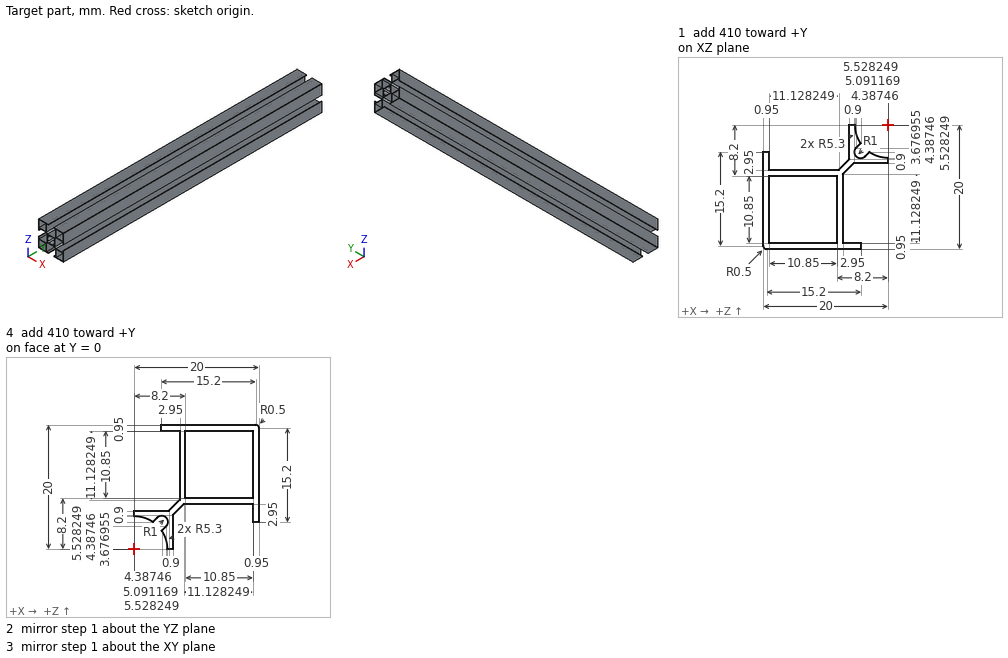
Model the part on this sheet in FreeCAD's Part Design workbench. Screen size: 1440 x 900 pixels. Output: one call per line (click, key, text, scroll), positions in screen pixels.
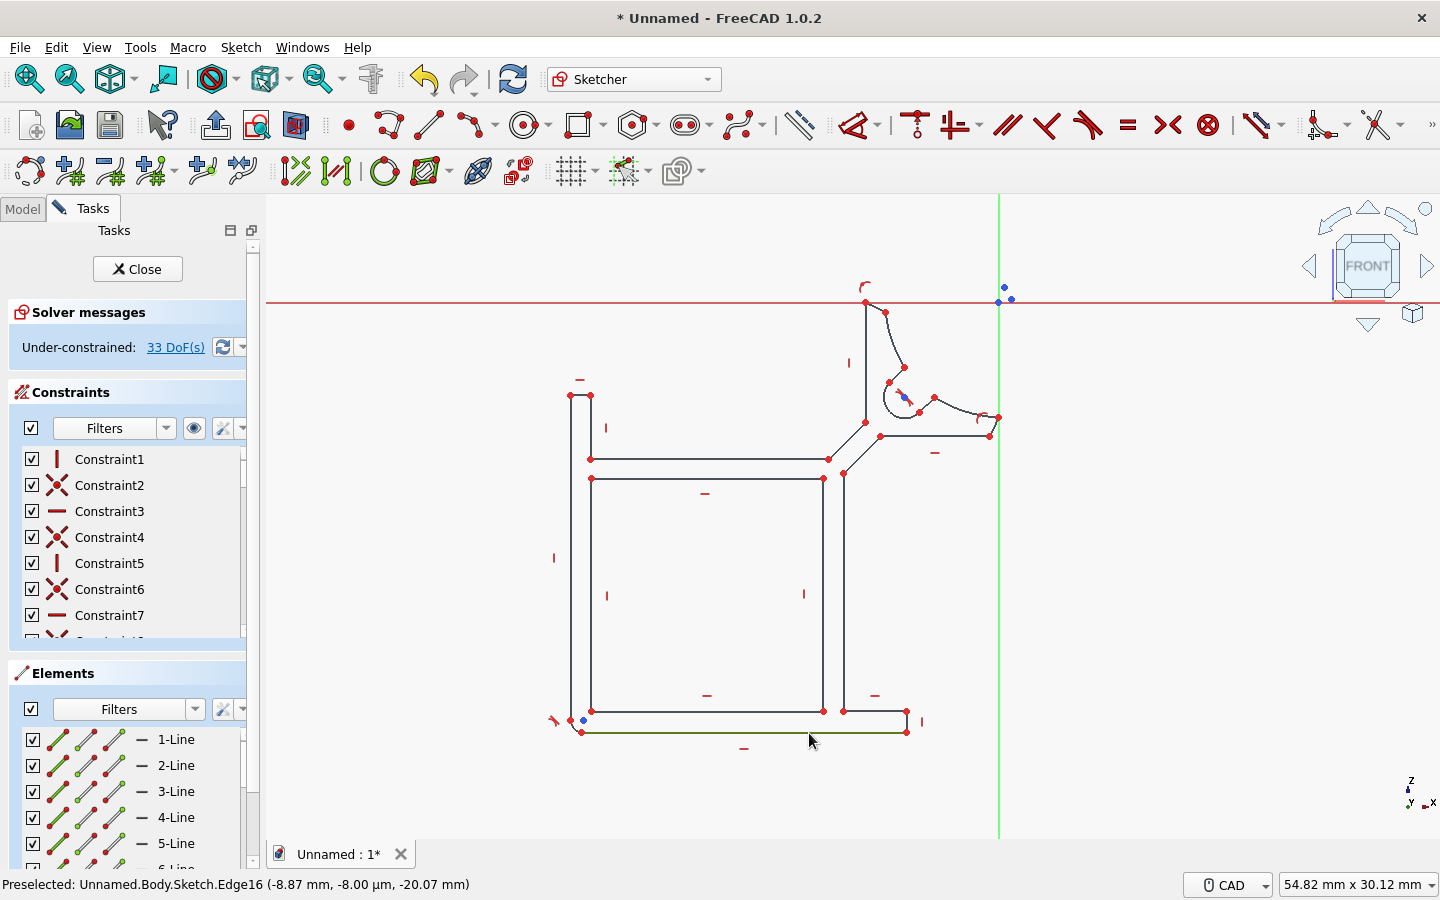
scroll(574, 728, up, 3)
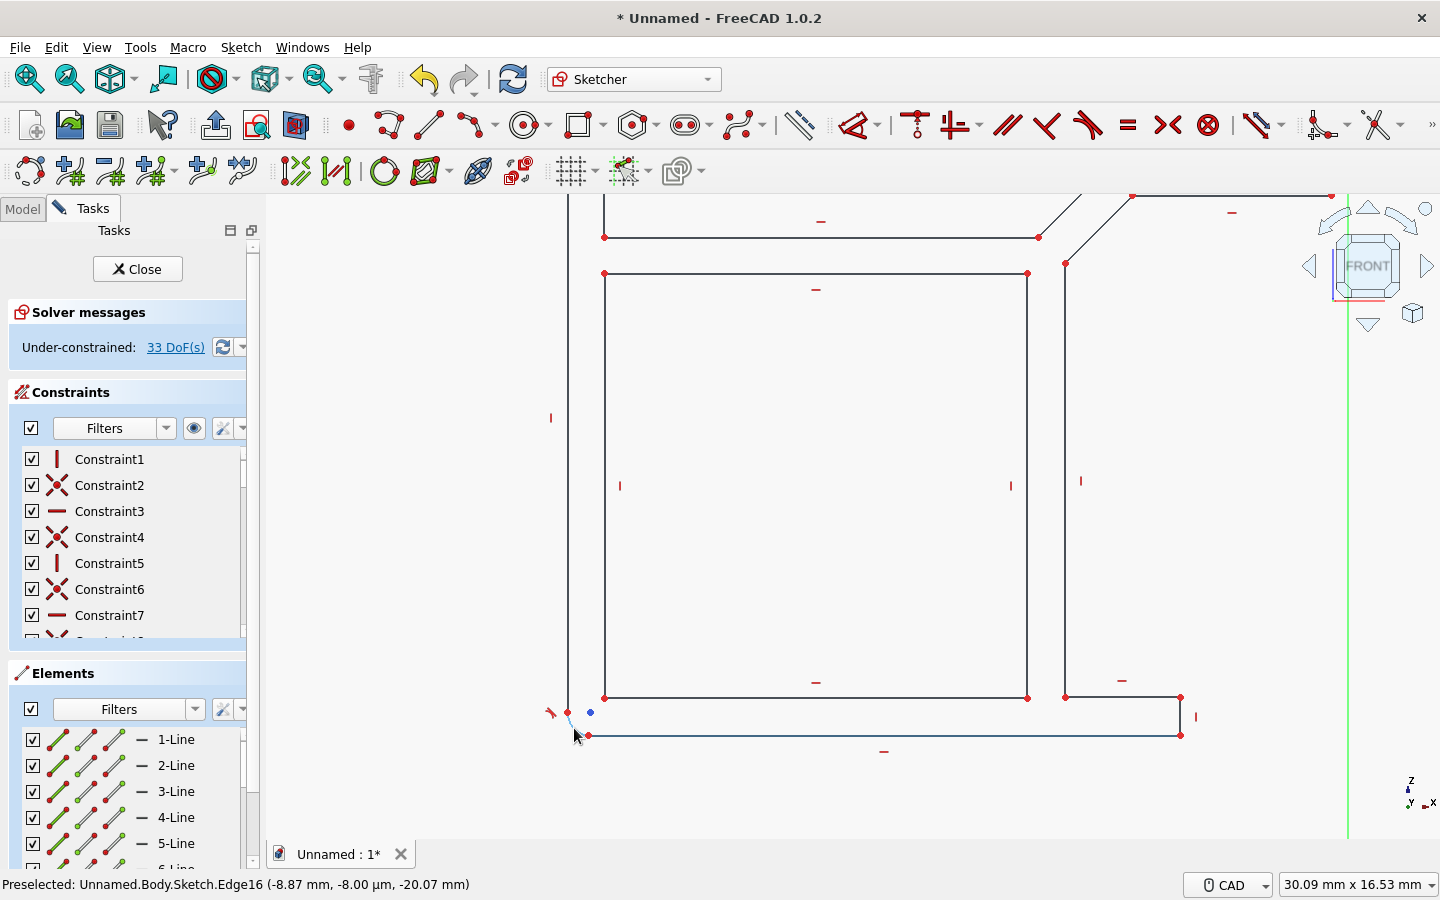
click(574, 728)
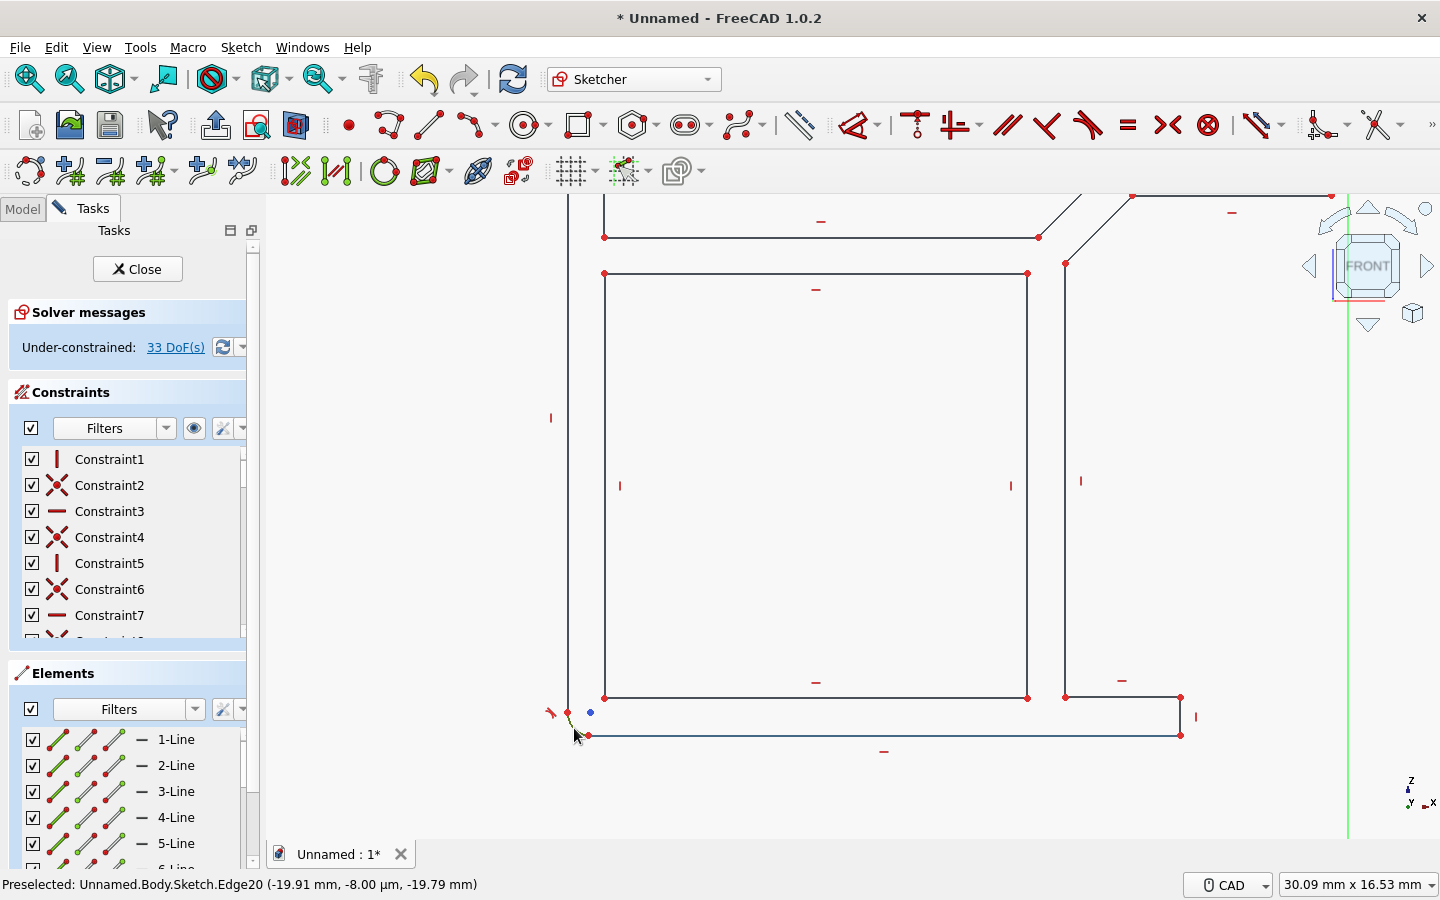
click(1088, 126)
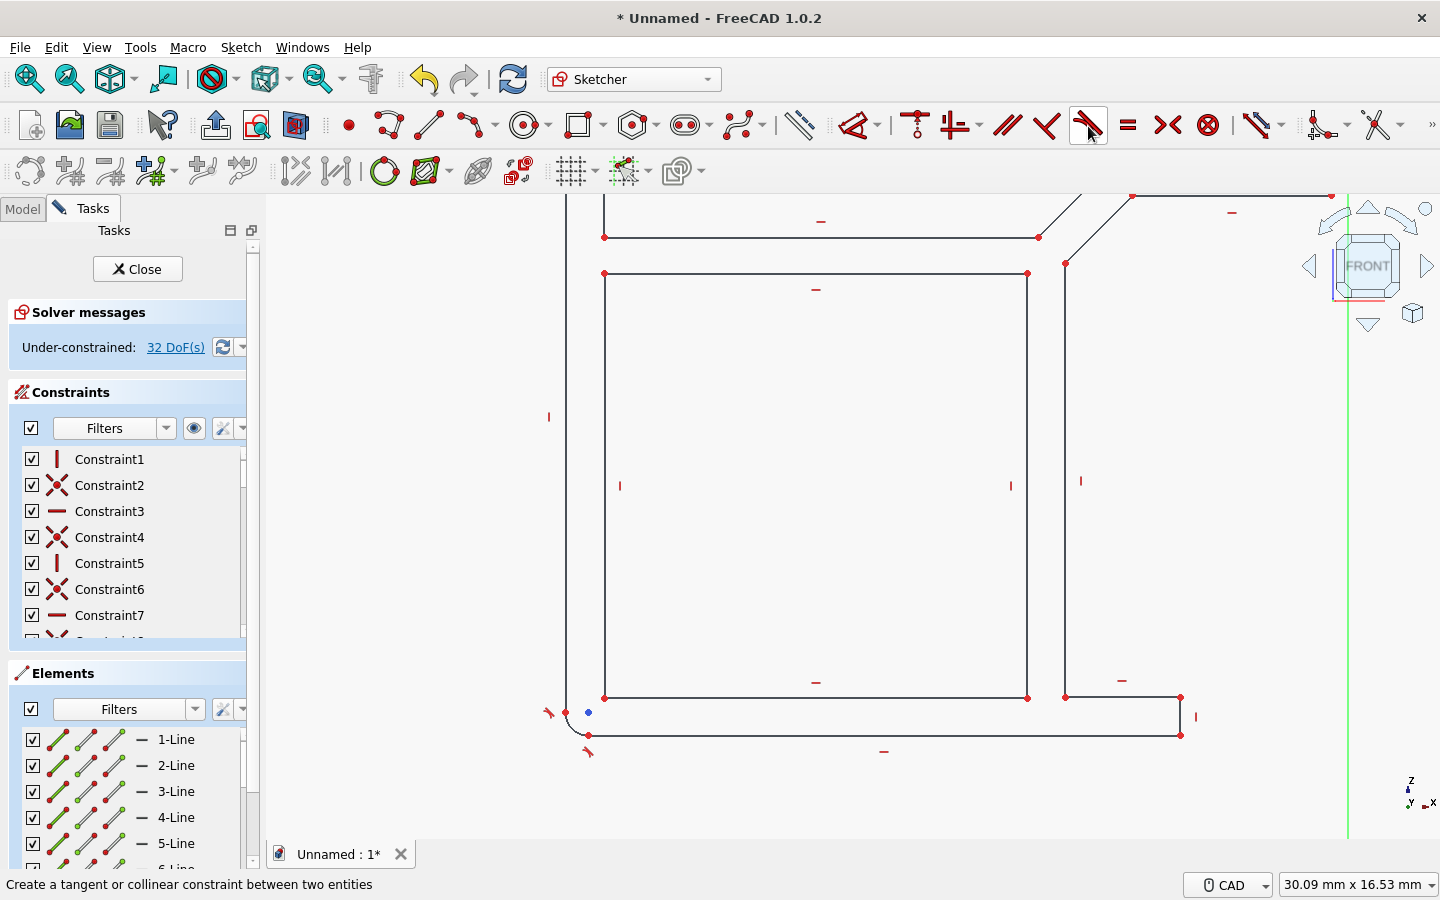
scroll(574, 728, down, 3)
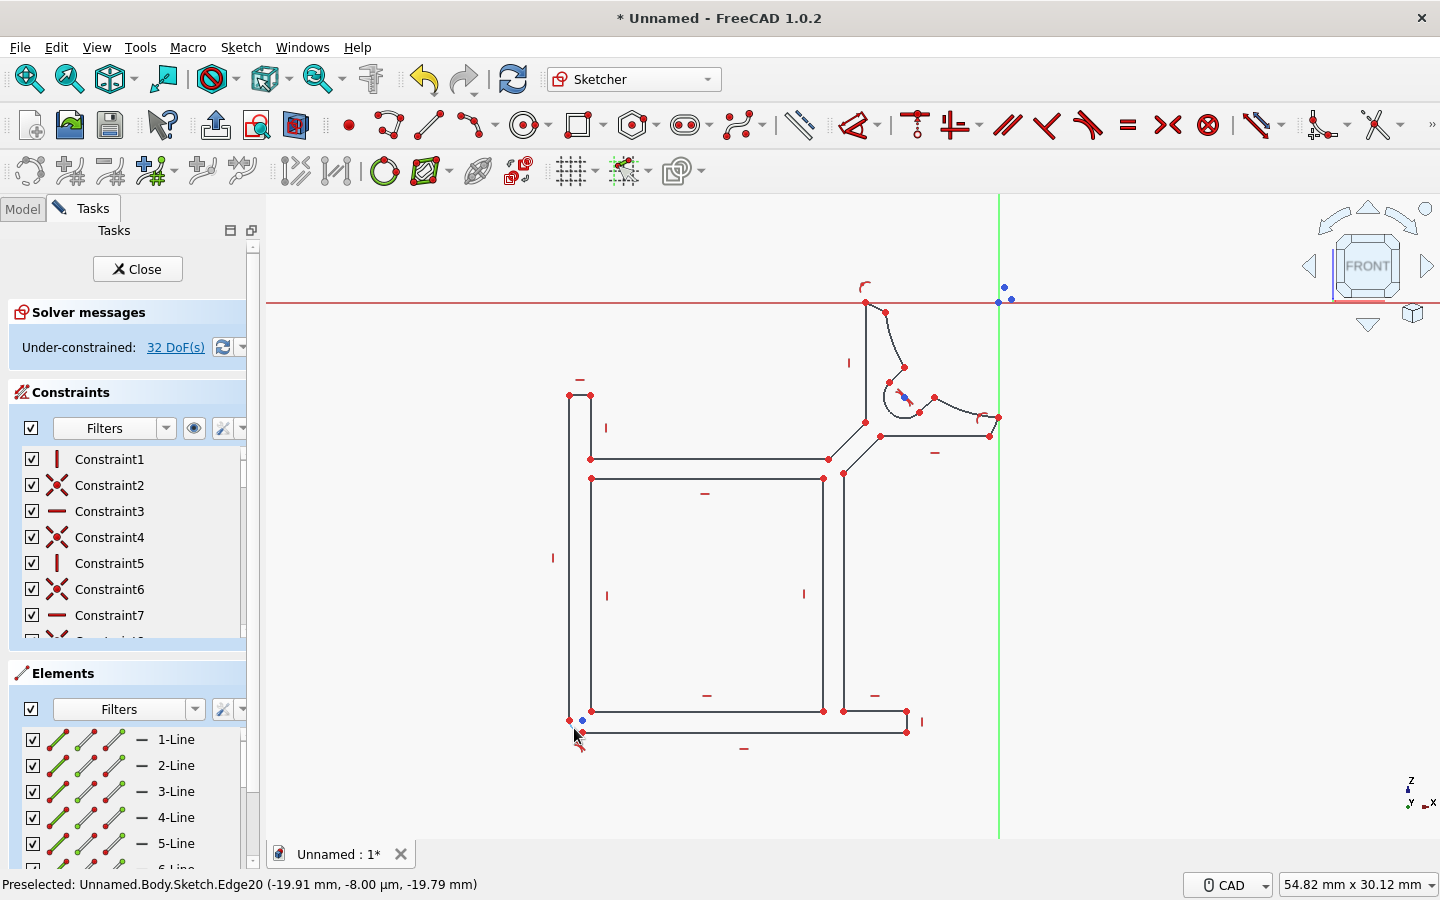
scroll(880, 309, up, 4)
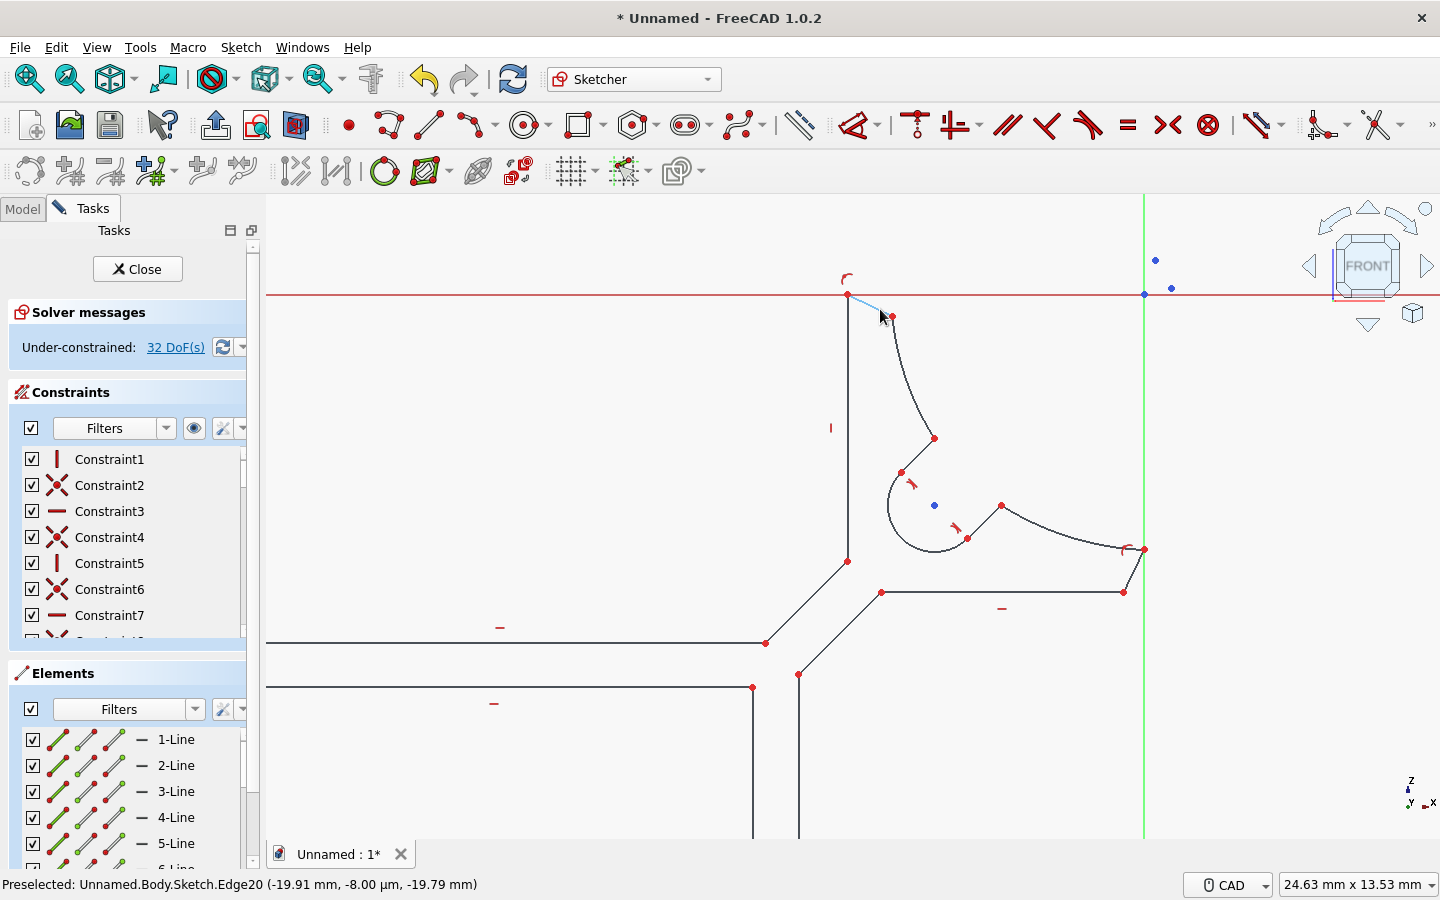
click(879, 310)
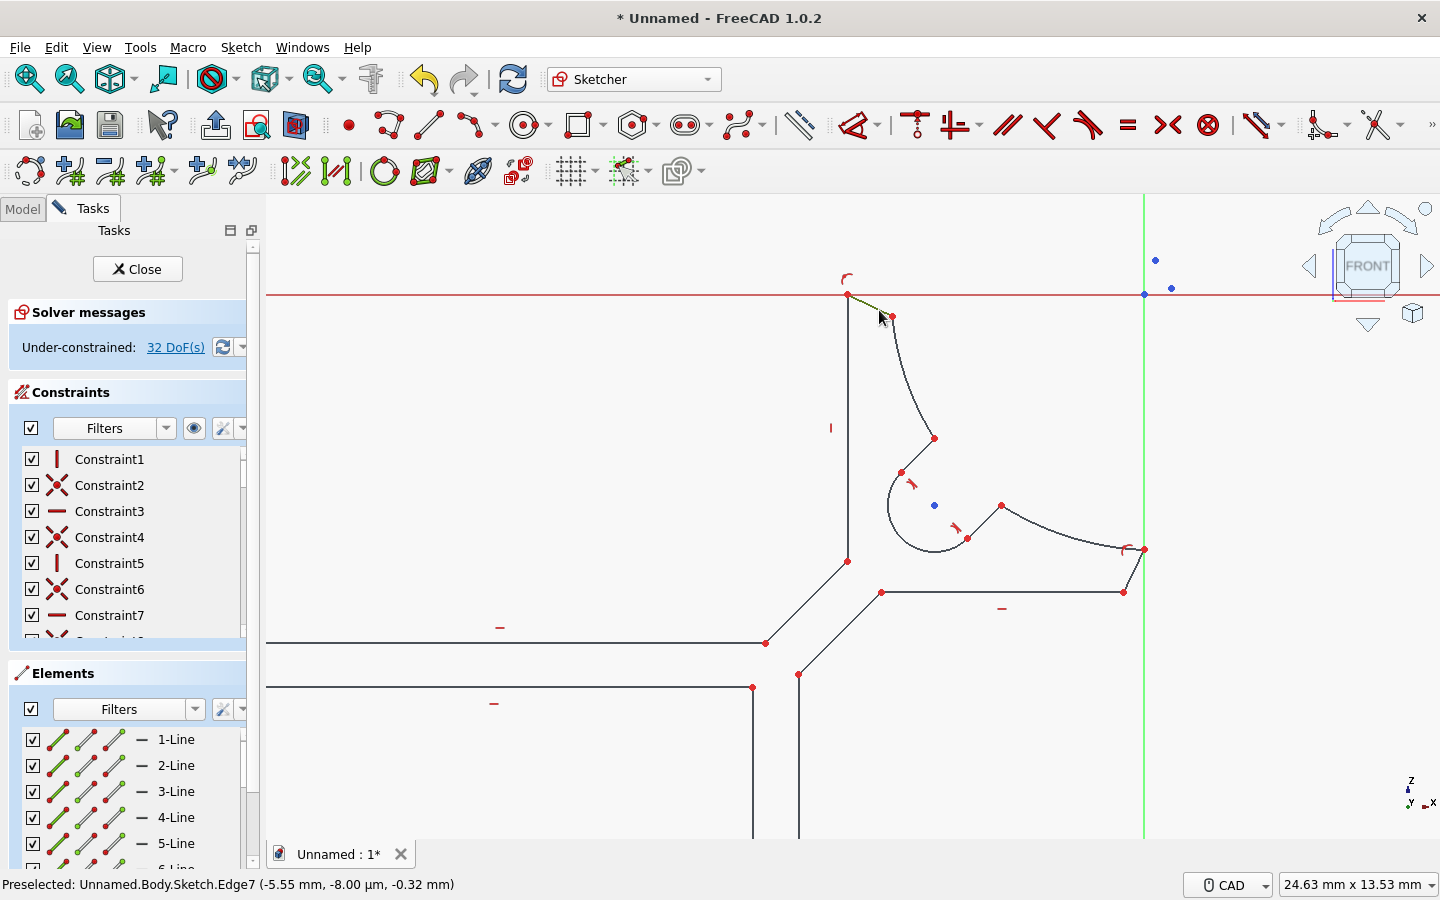
key(h)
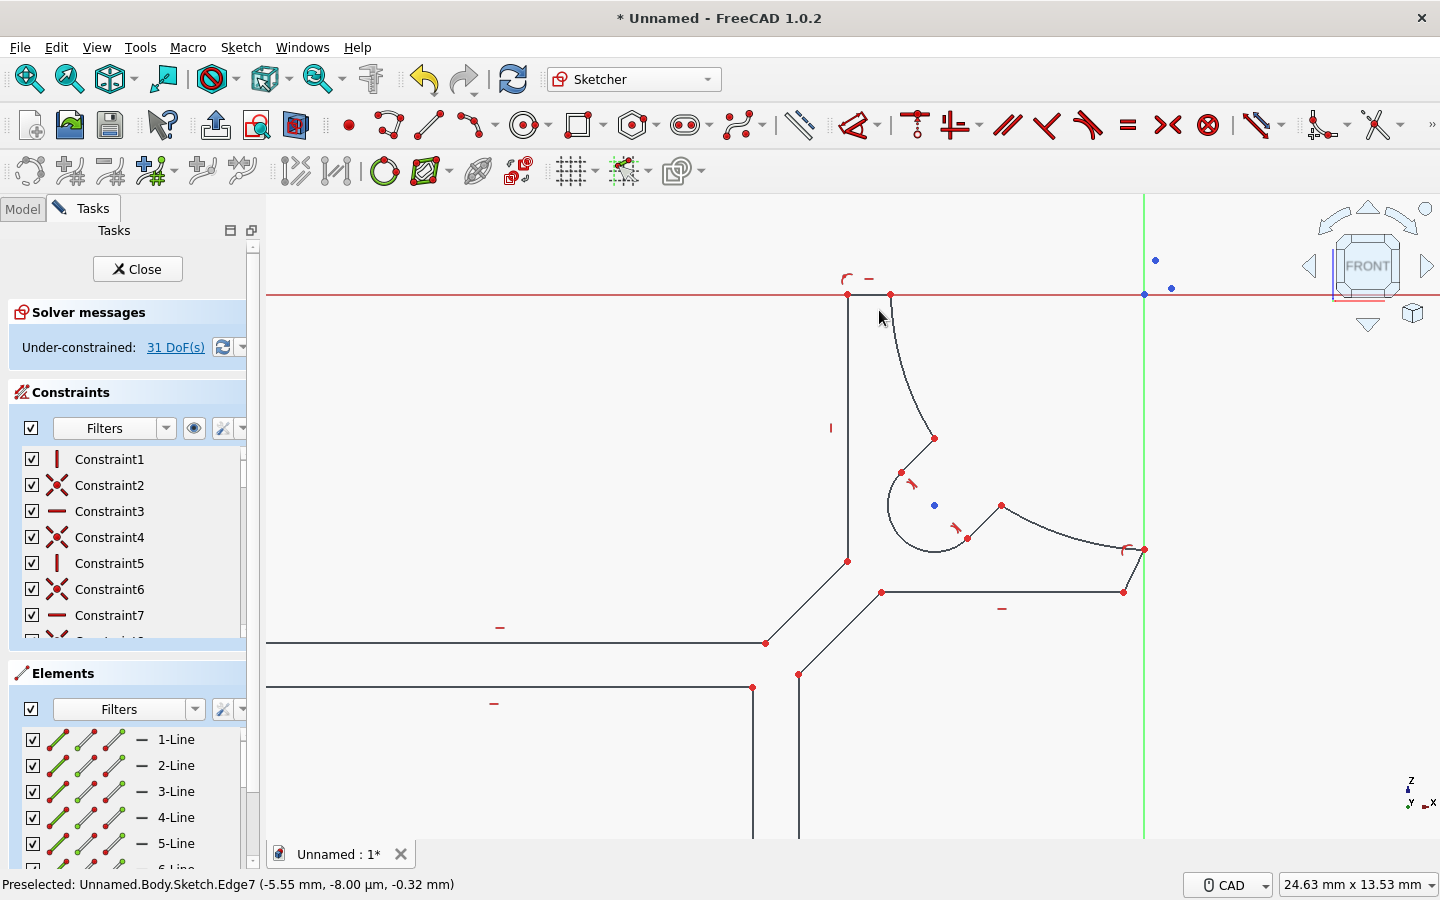
click(1130, 580)